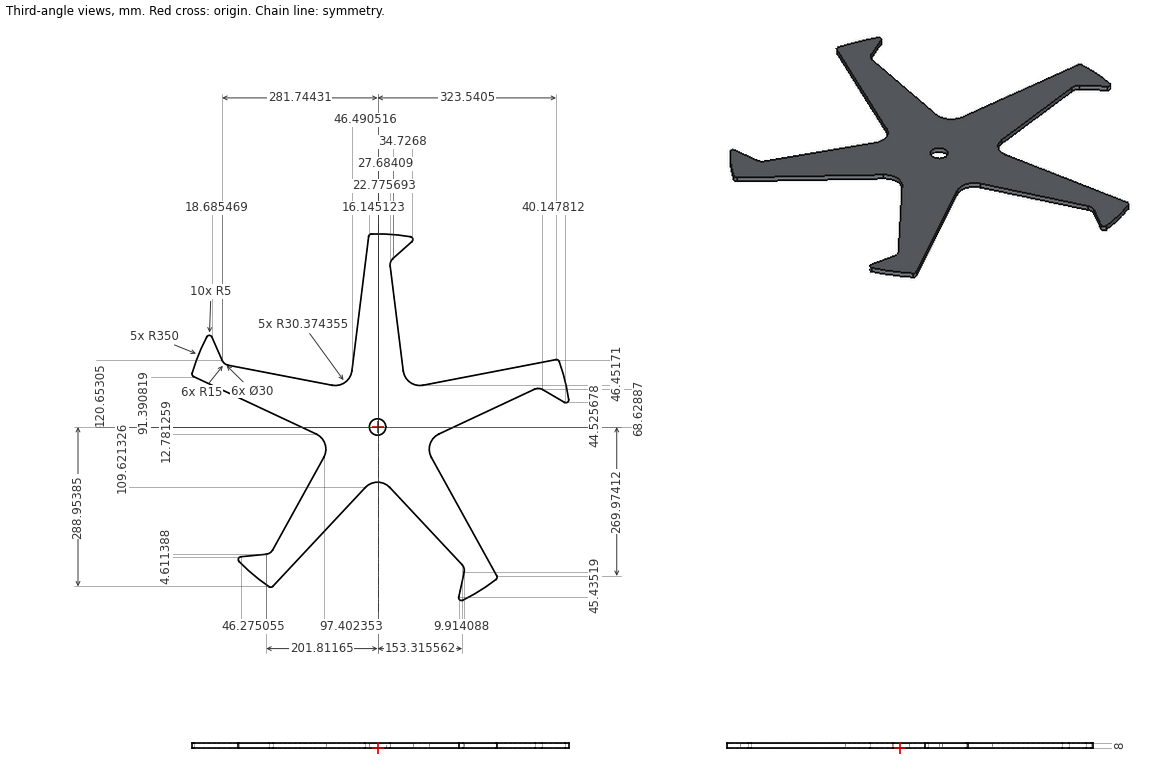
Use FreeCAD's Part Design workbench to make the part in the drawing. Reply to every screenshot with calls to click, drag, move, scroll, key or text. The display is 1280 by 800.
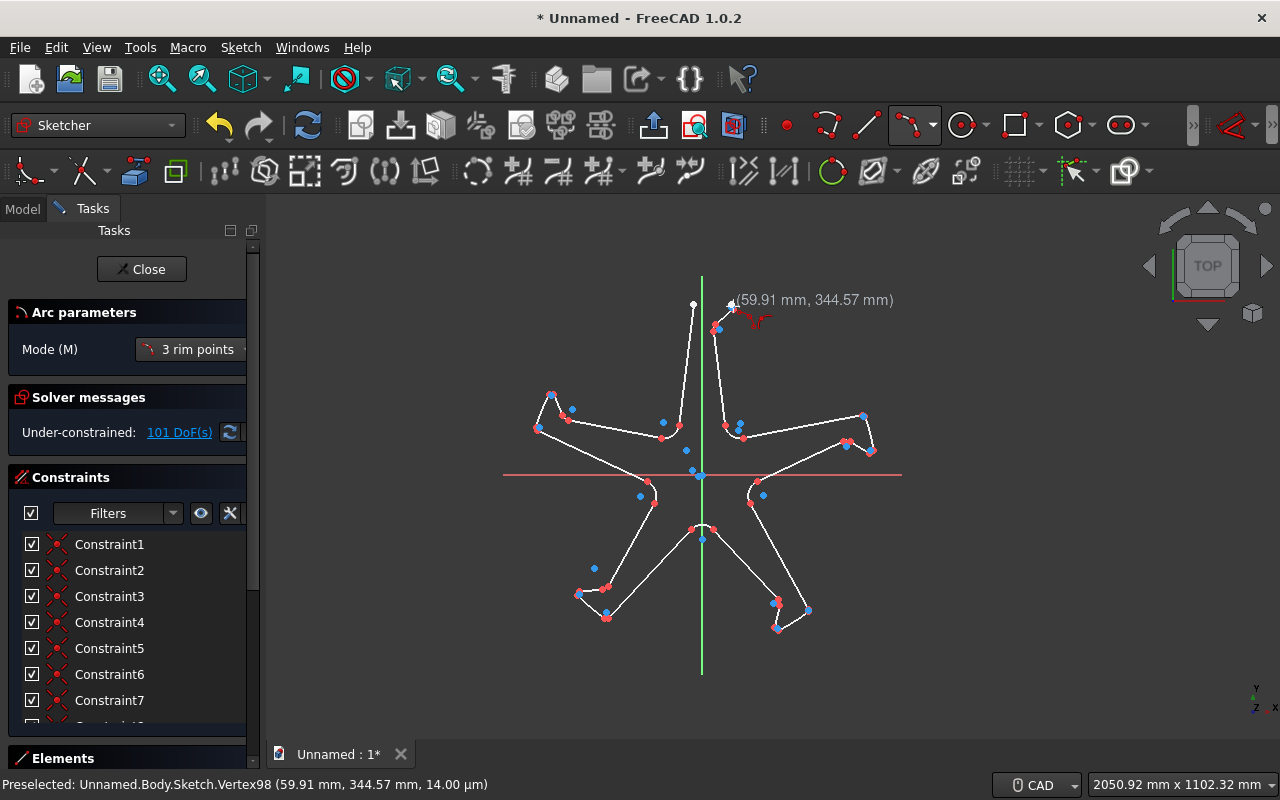
scroll(697, 302, up, 8)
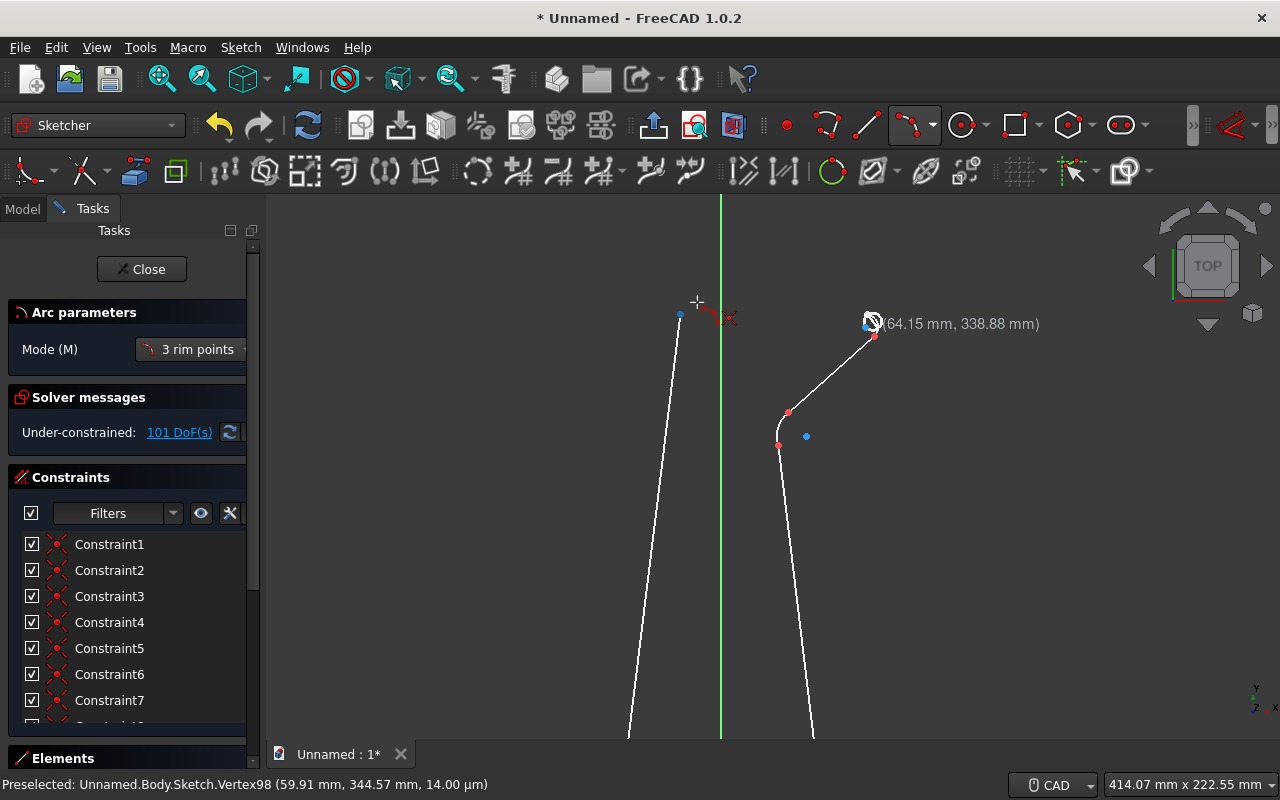
click(693, 302)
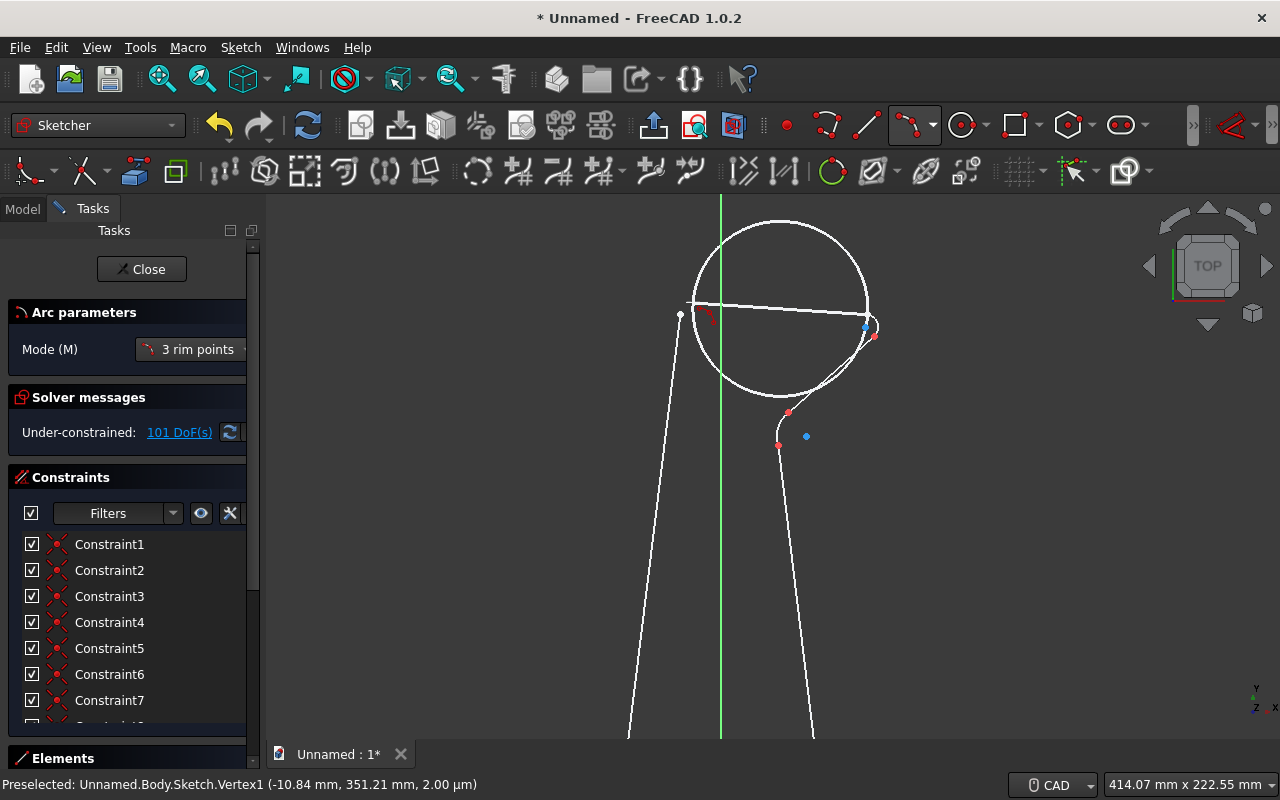
scroll(781, 303, up, 7)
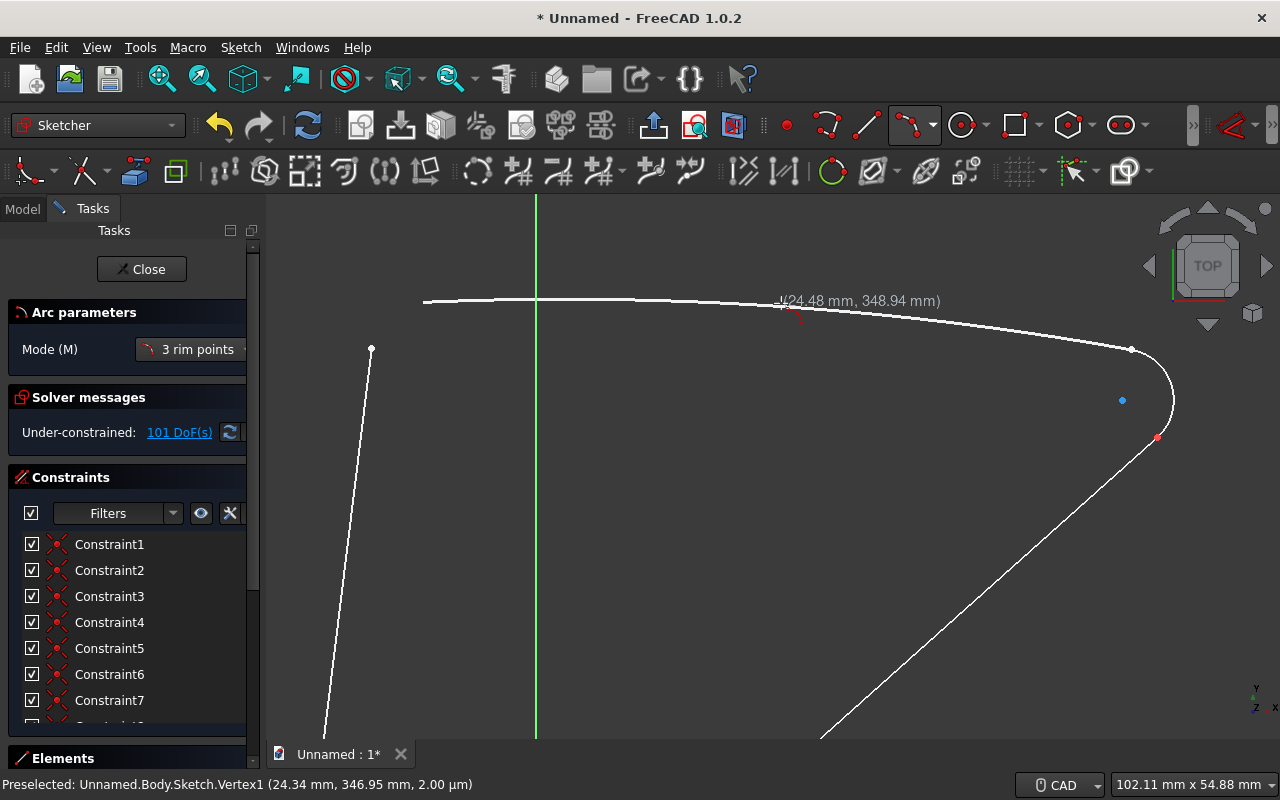
click(779, 304)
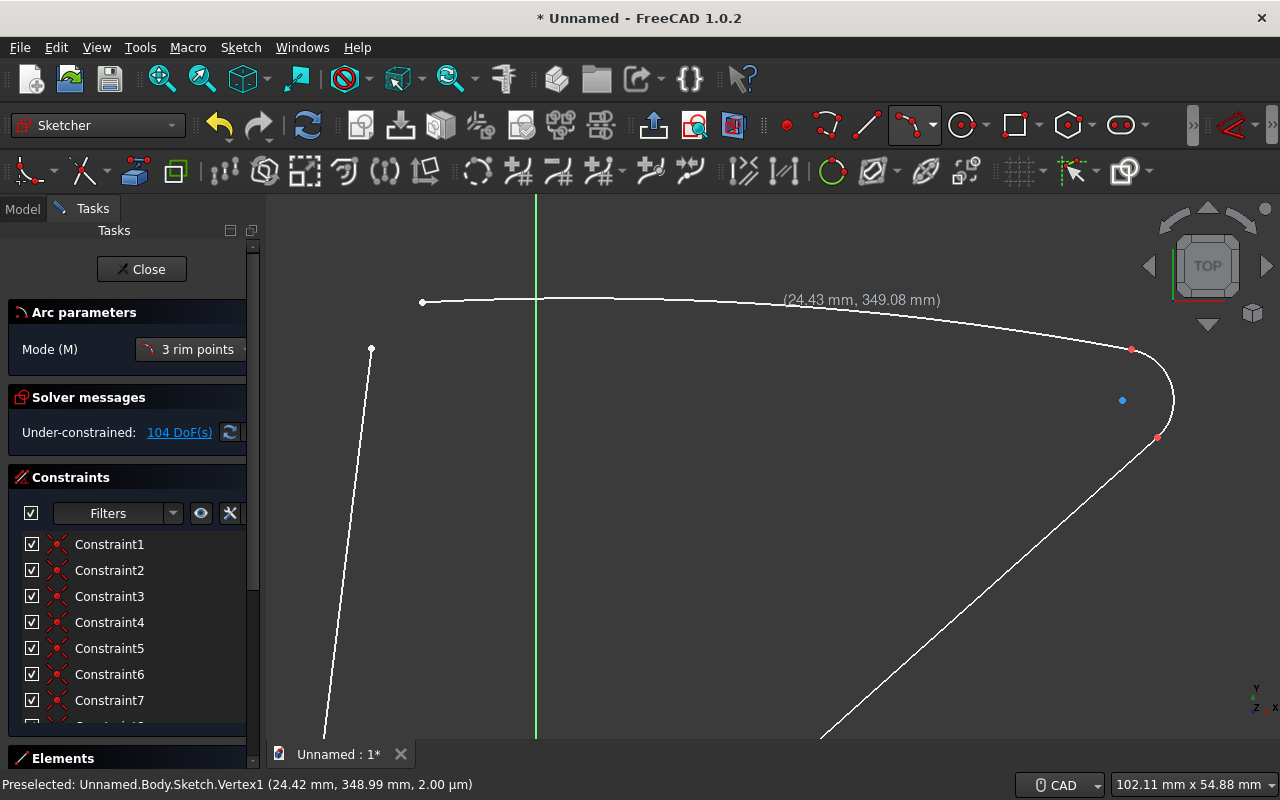
scroll(711, 303, down, 15)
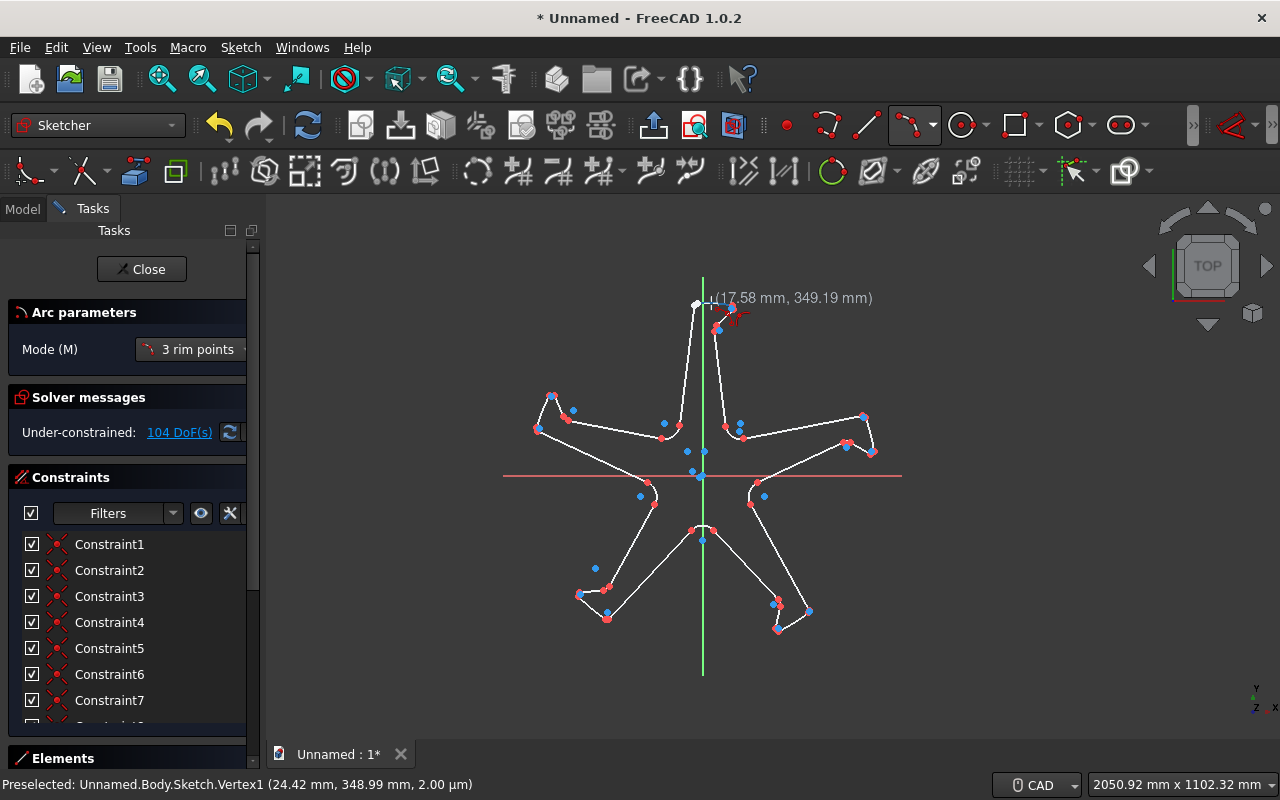
scroll(697, 303, up, 8)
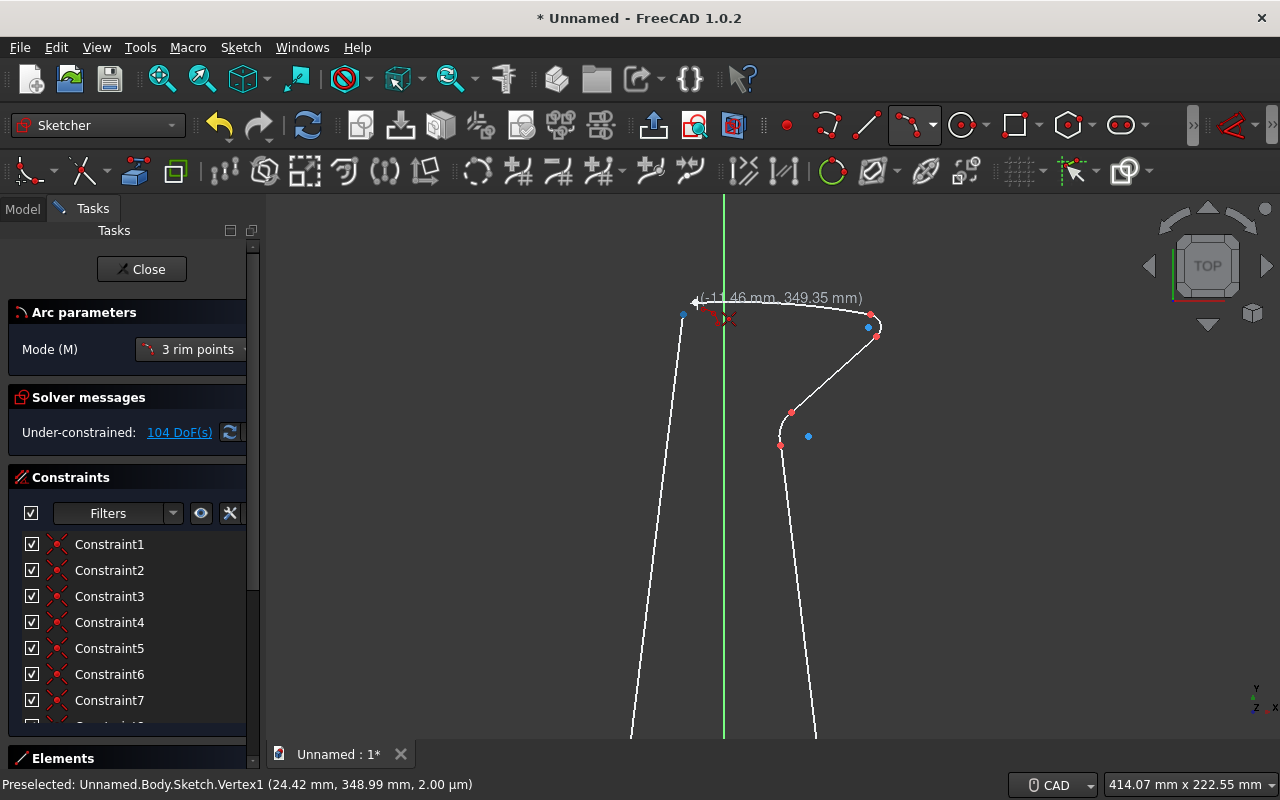
click(696, 303)
click(683, 314)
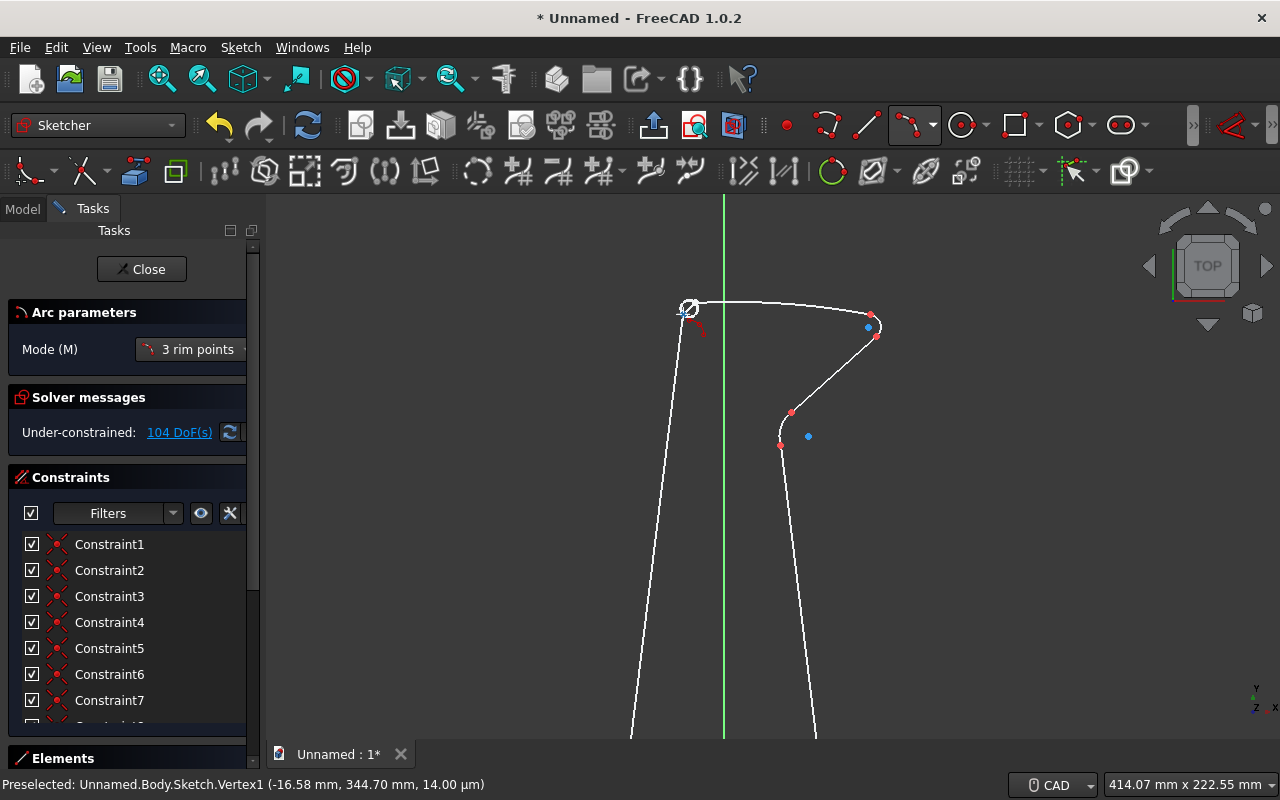
scroll(688, 305, up, 9)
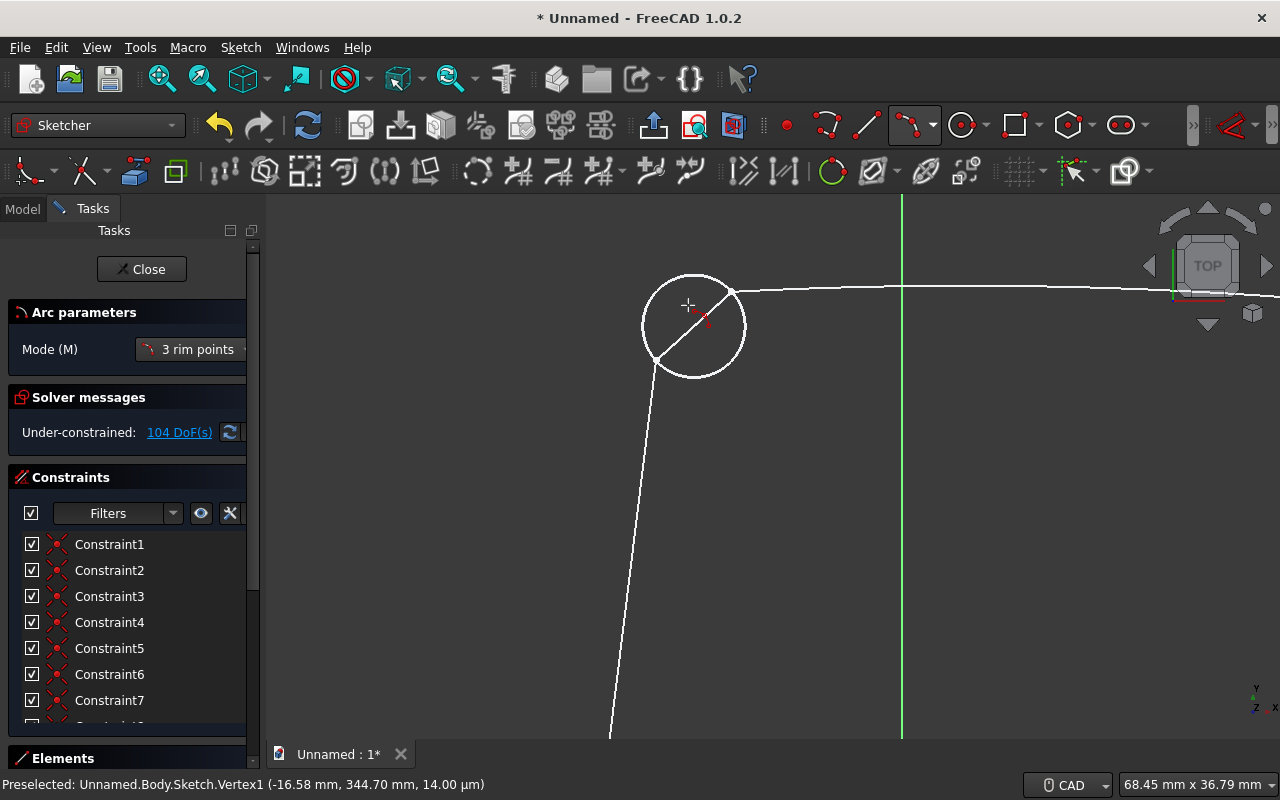
click(686, 304)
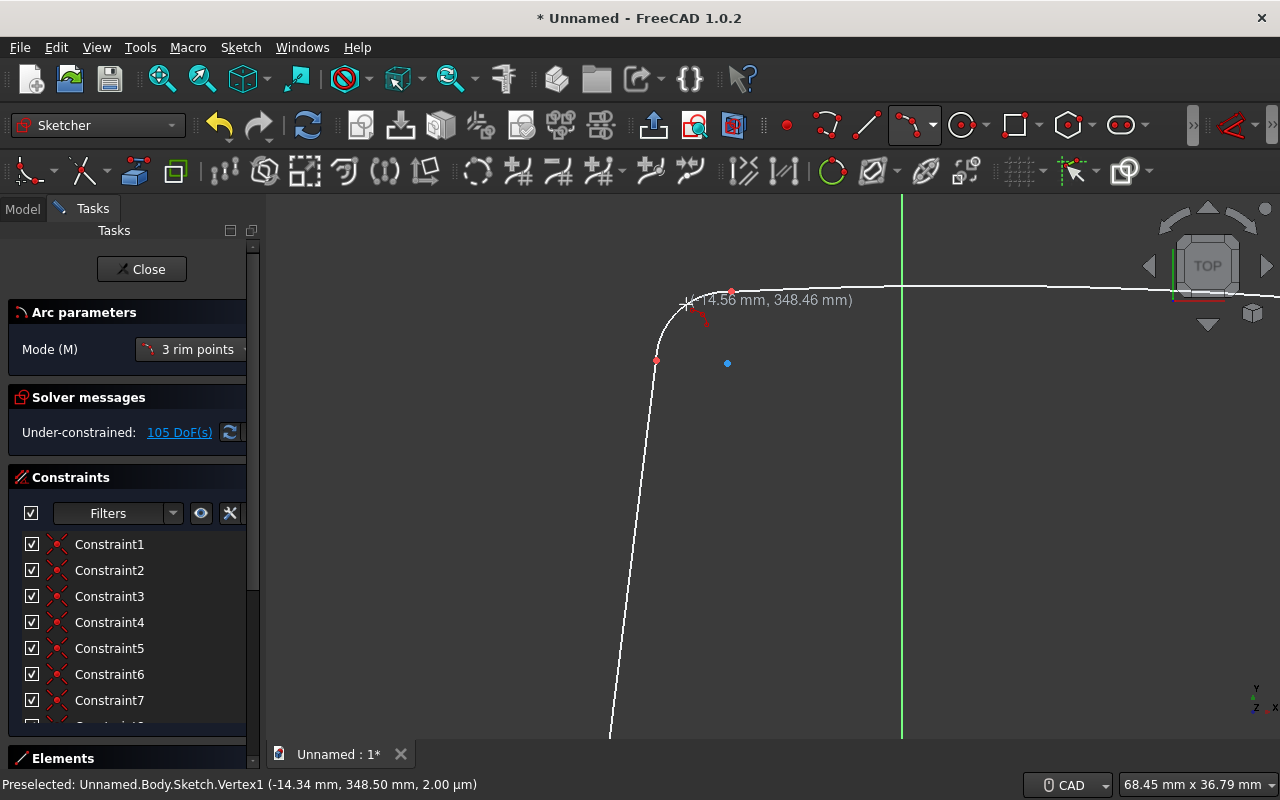
click(962, 126)